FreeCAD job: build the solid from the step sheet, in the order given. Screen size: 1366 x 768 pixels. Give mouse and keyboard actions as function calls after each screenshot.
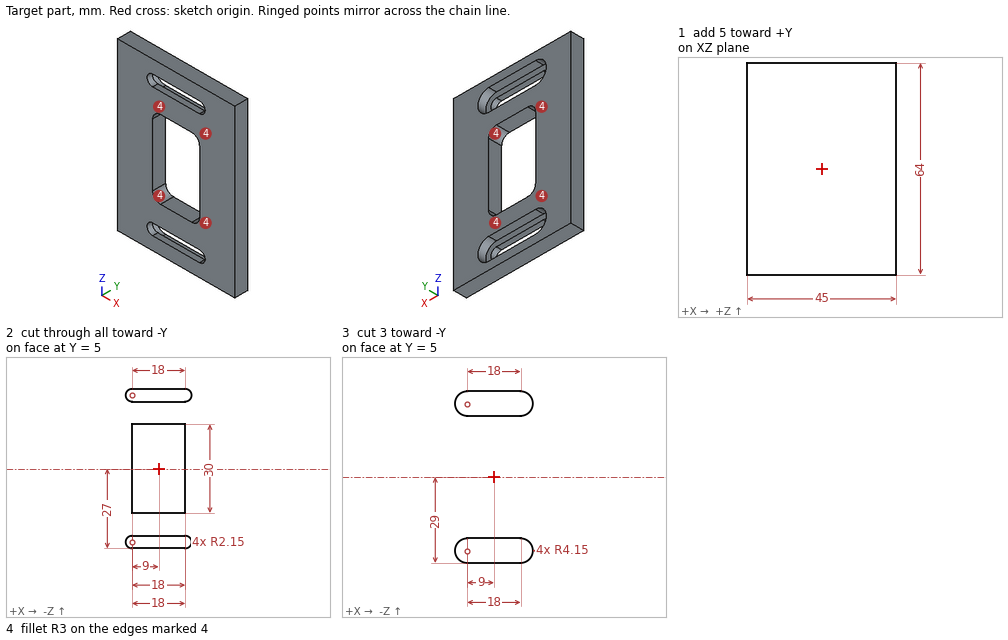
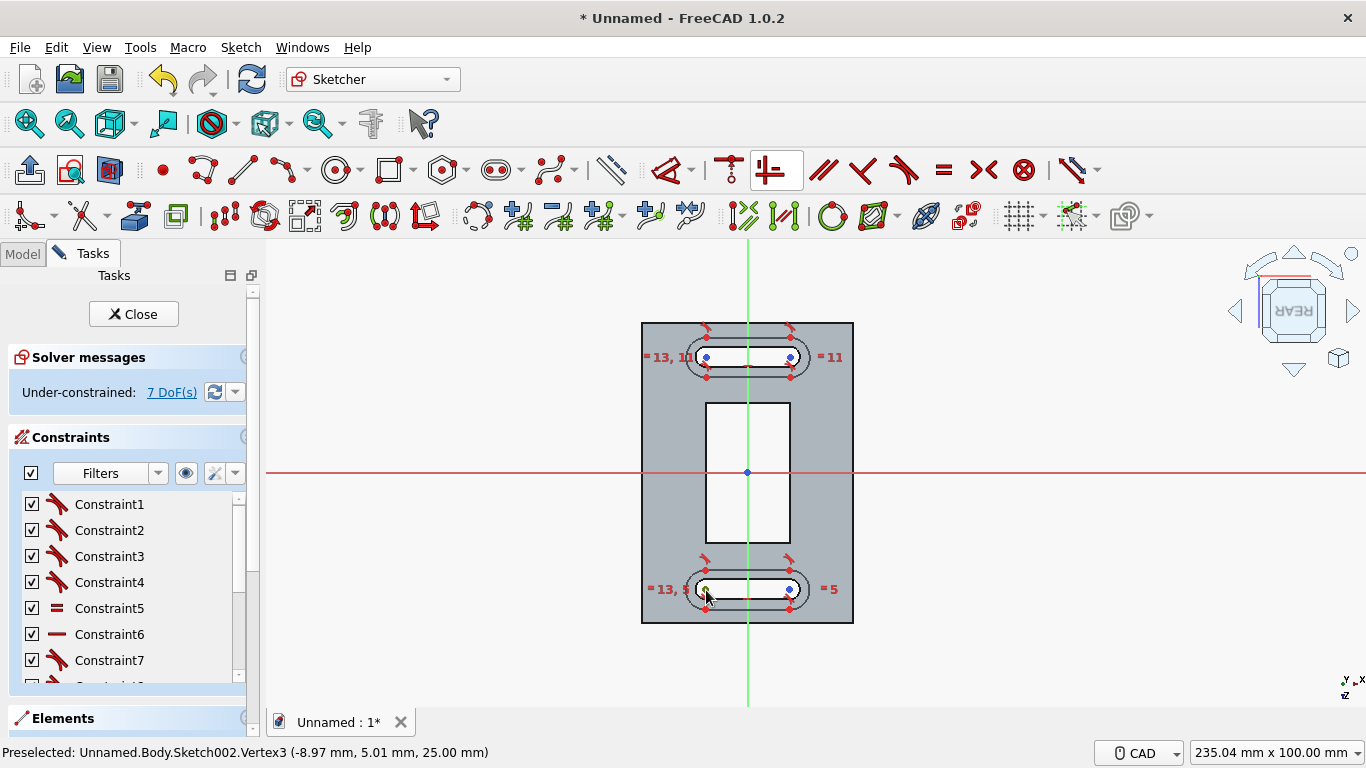
click(706, 358)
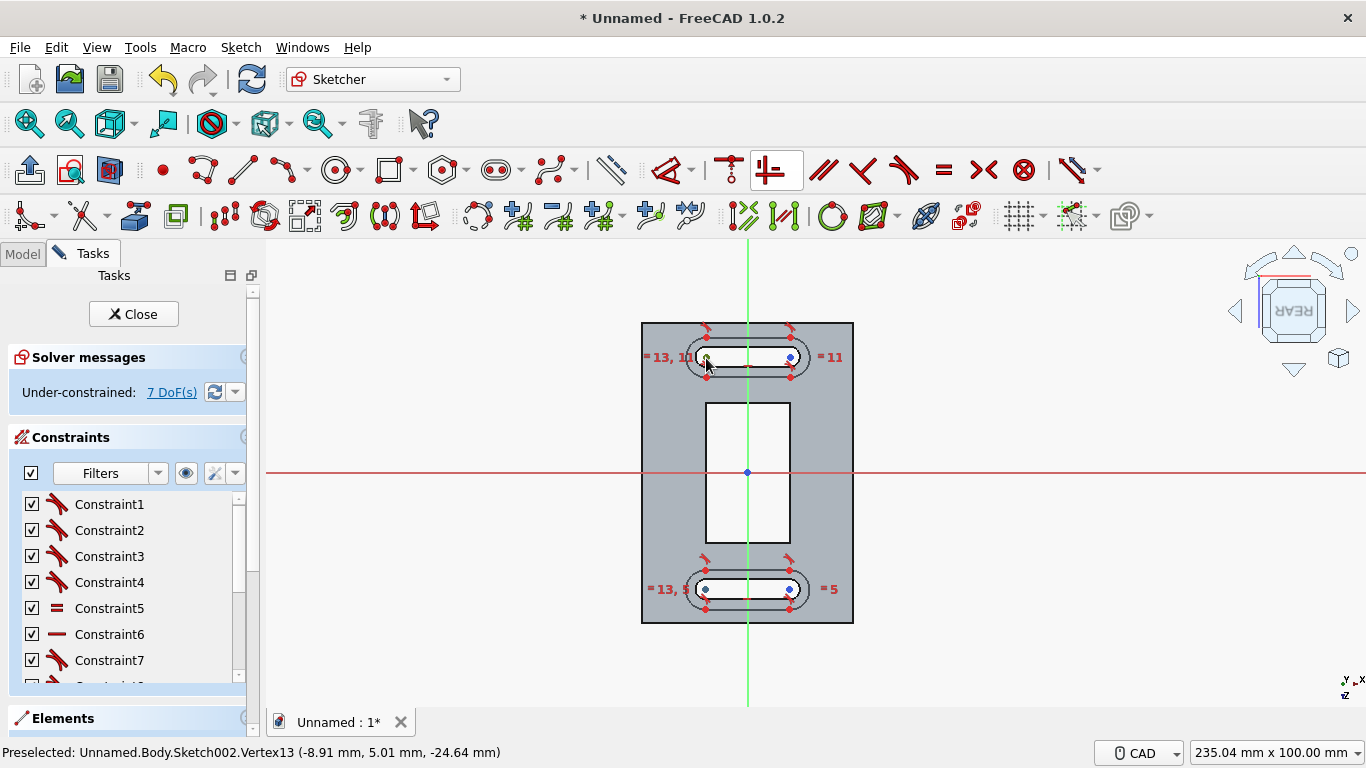
click(359, 473)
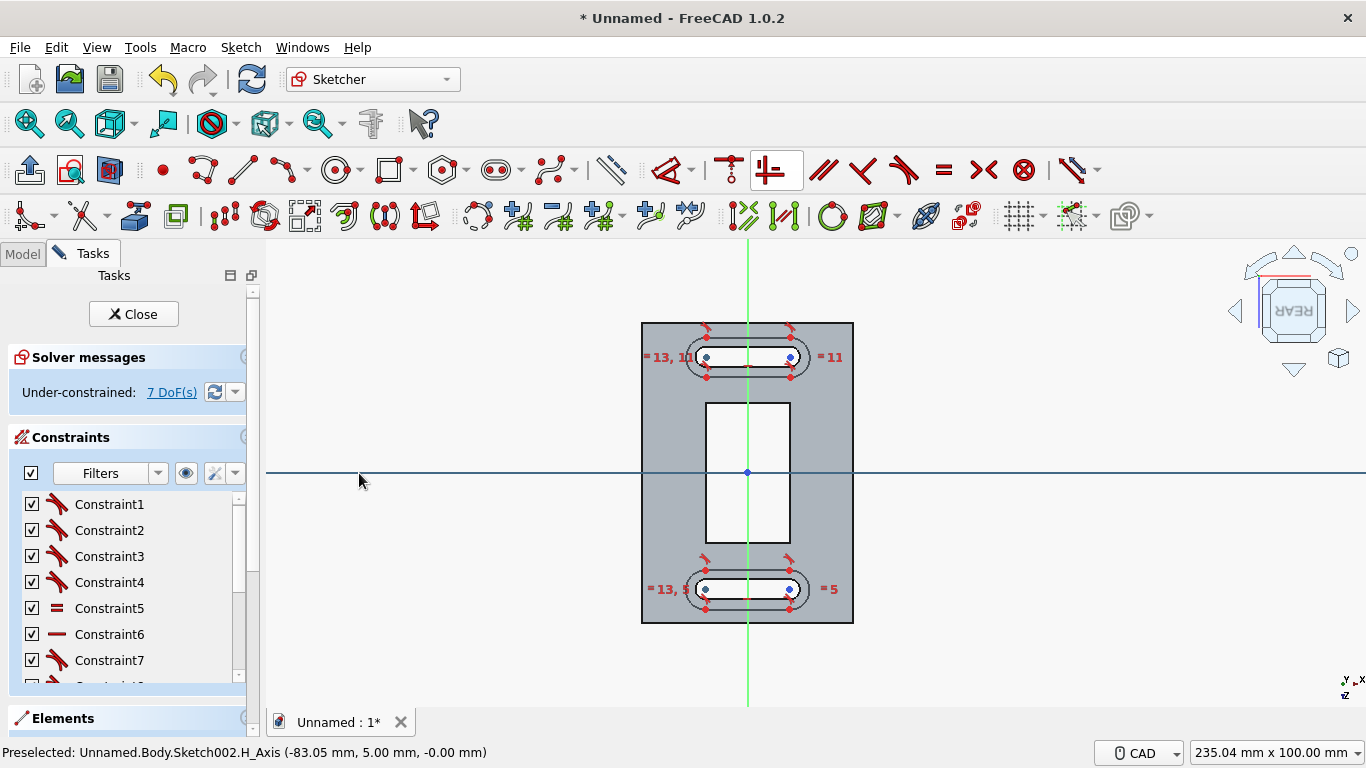
click(984, 170)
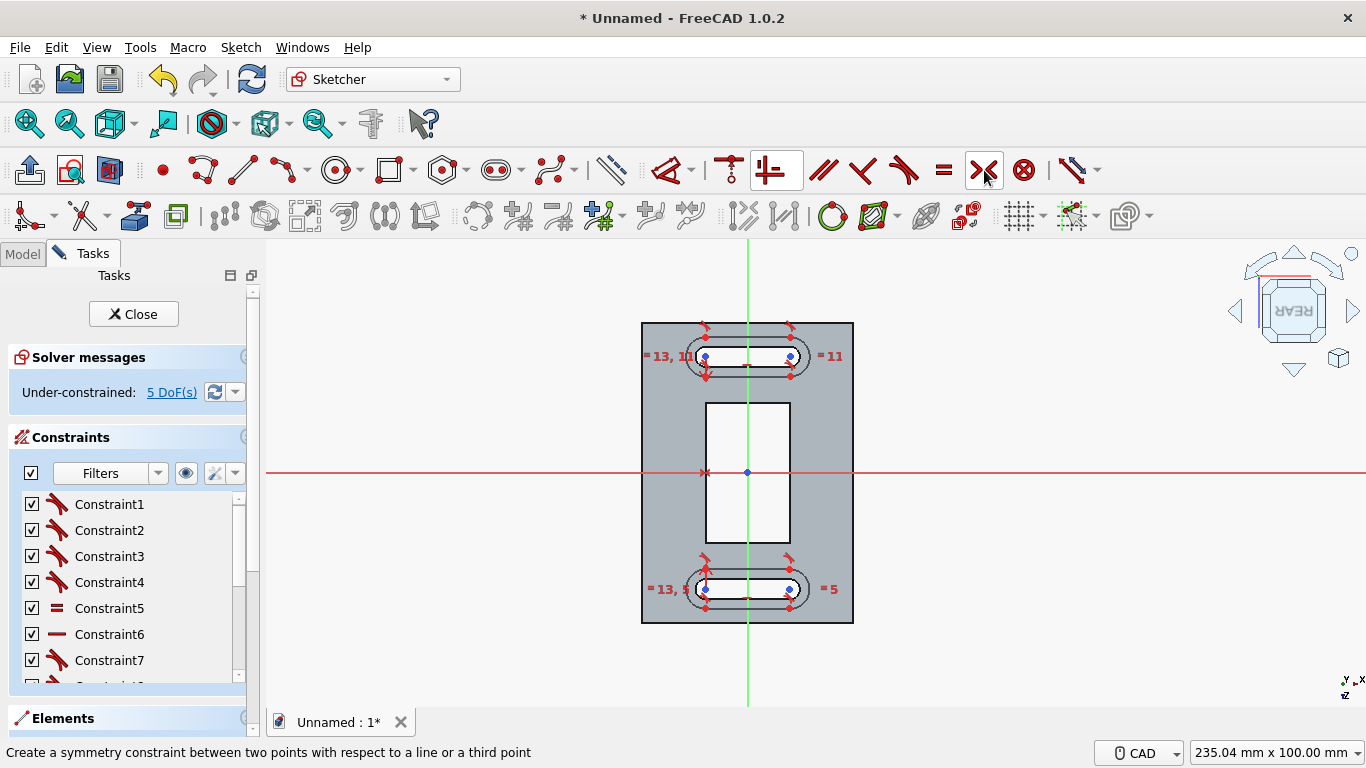
click(666, 170)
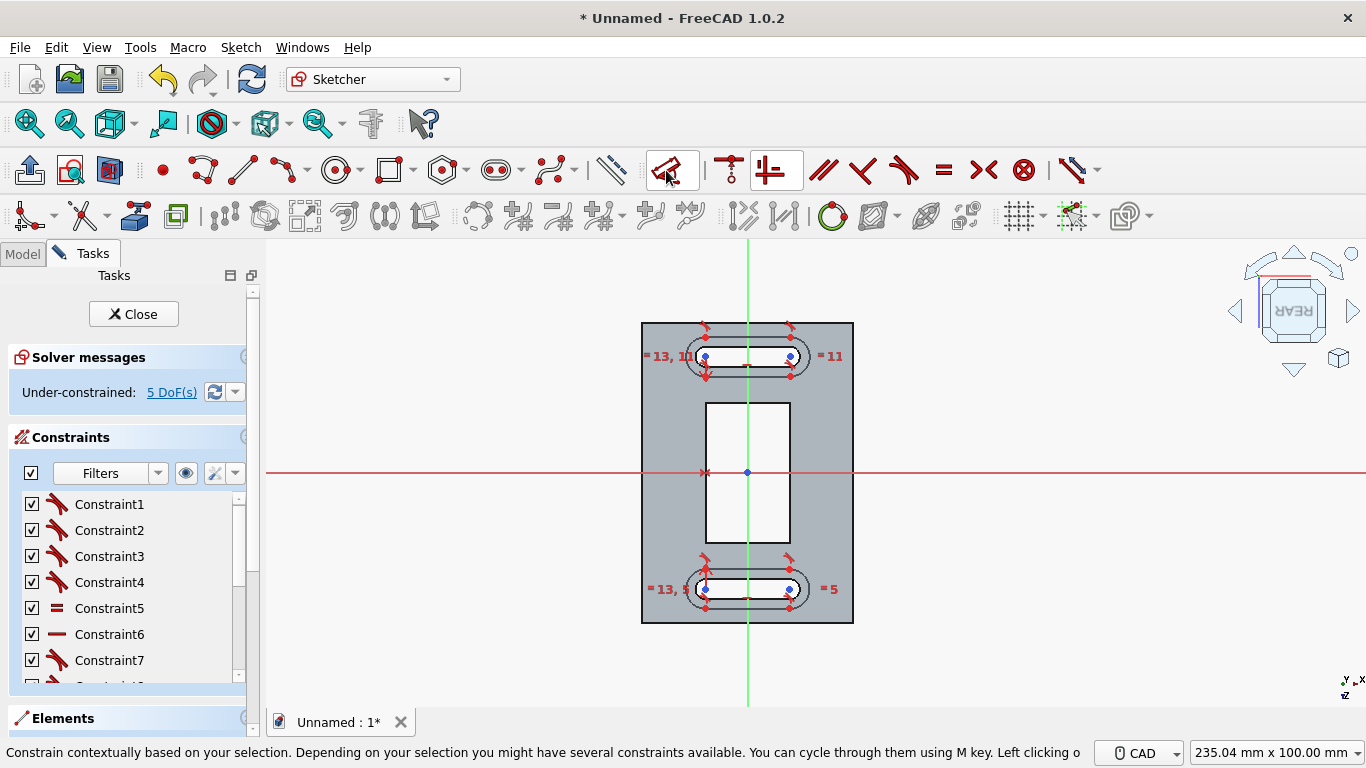
scroll(690, 578, up, 4)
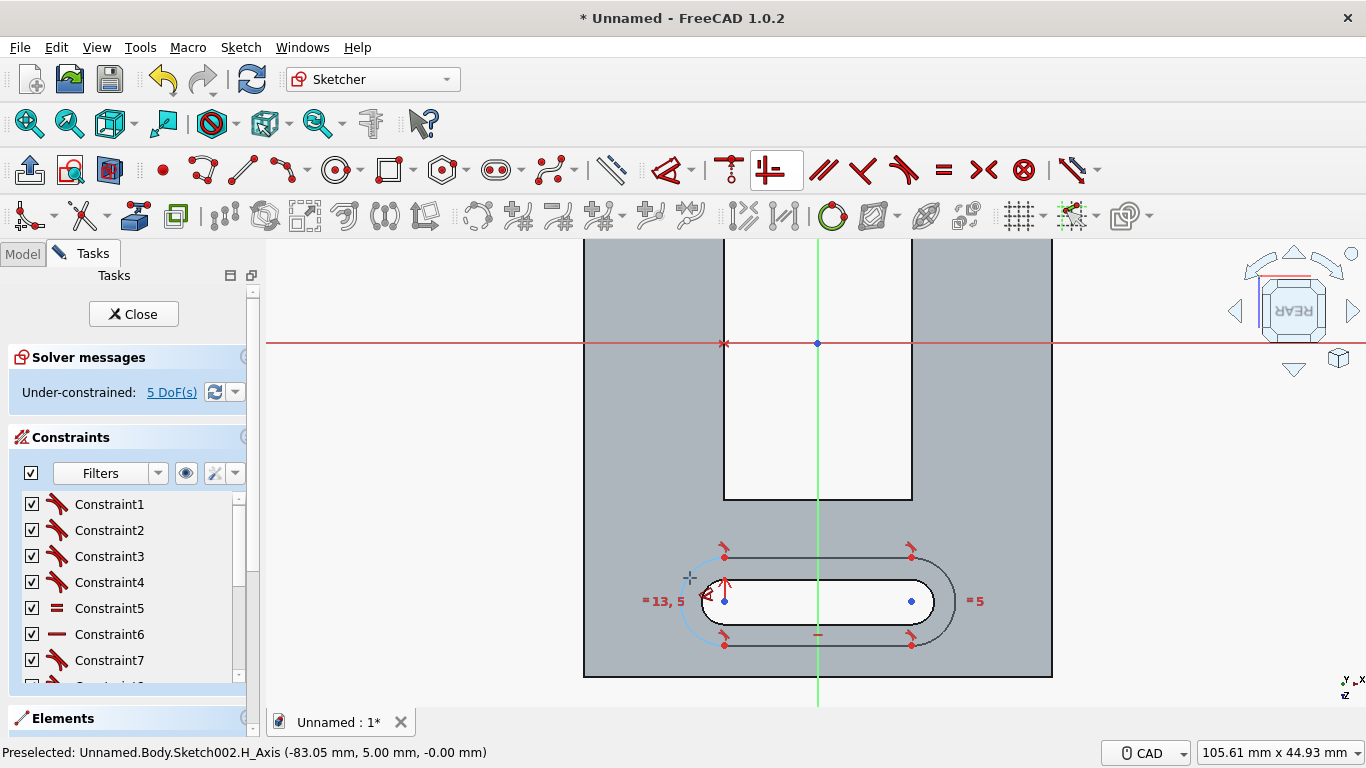
click(689, 576)
click(663, 557)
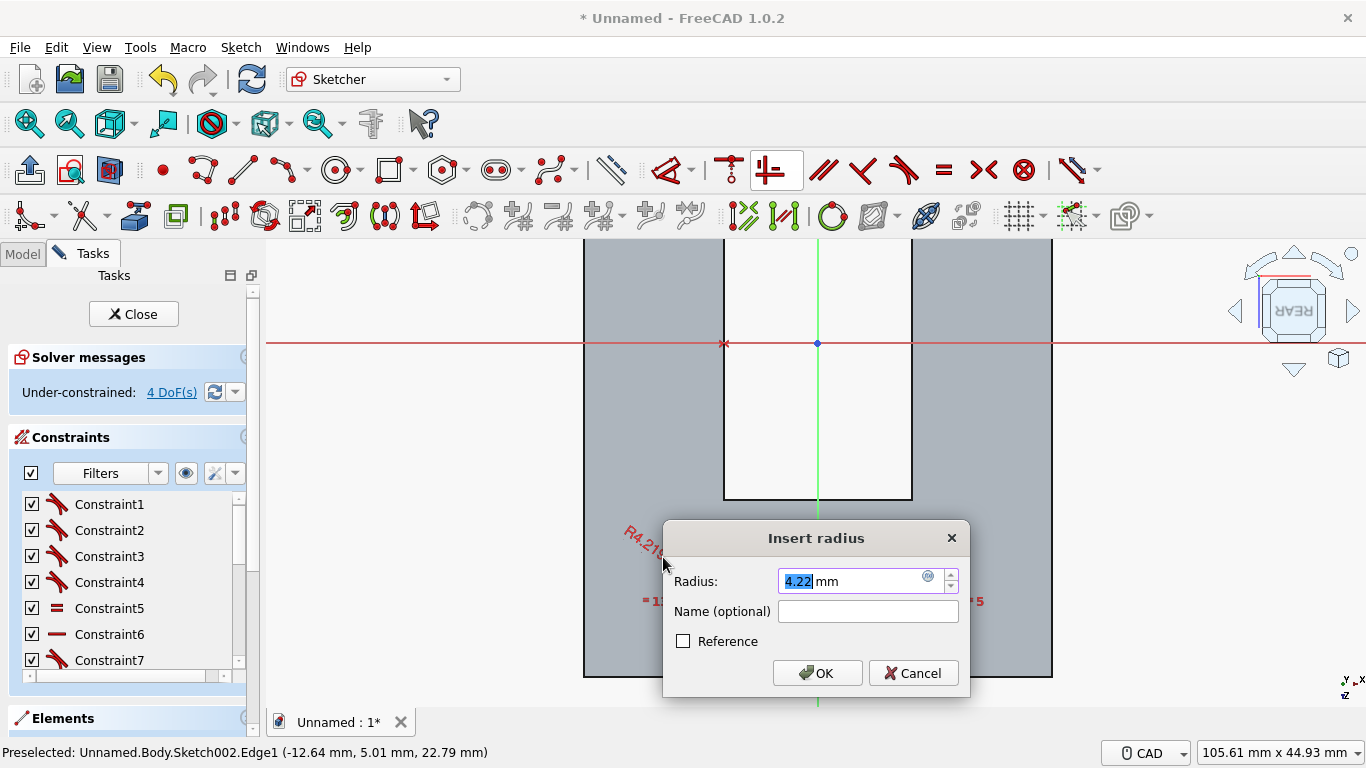
text(4.15)
key(Return)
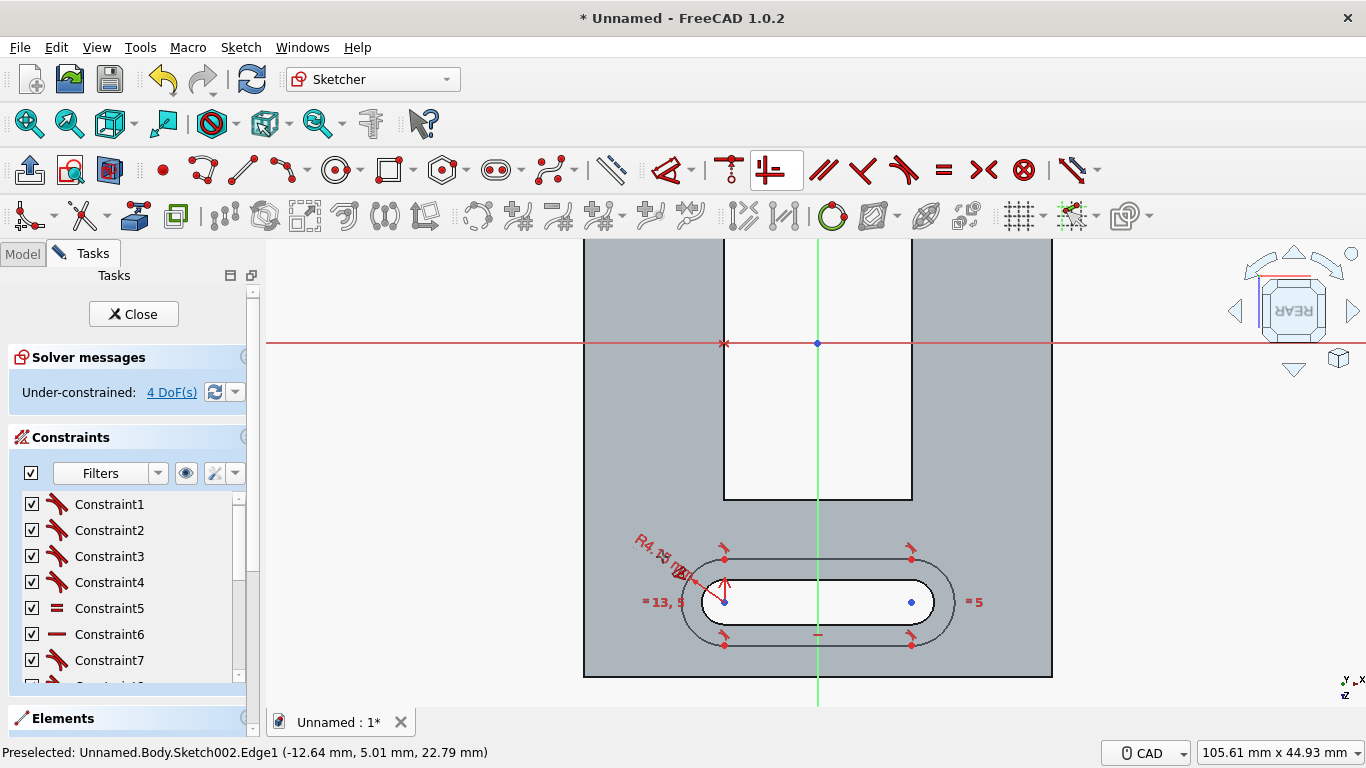
click(781, 559)
click(775, 593)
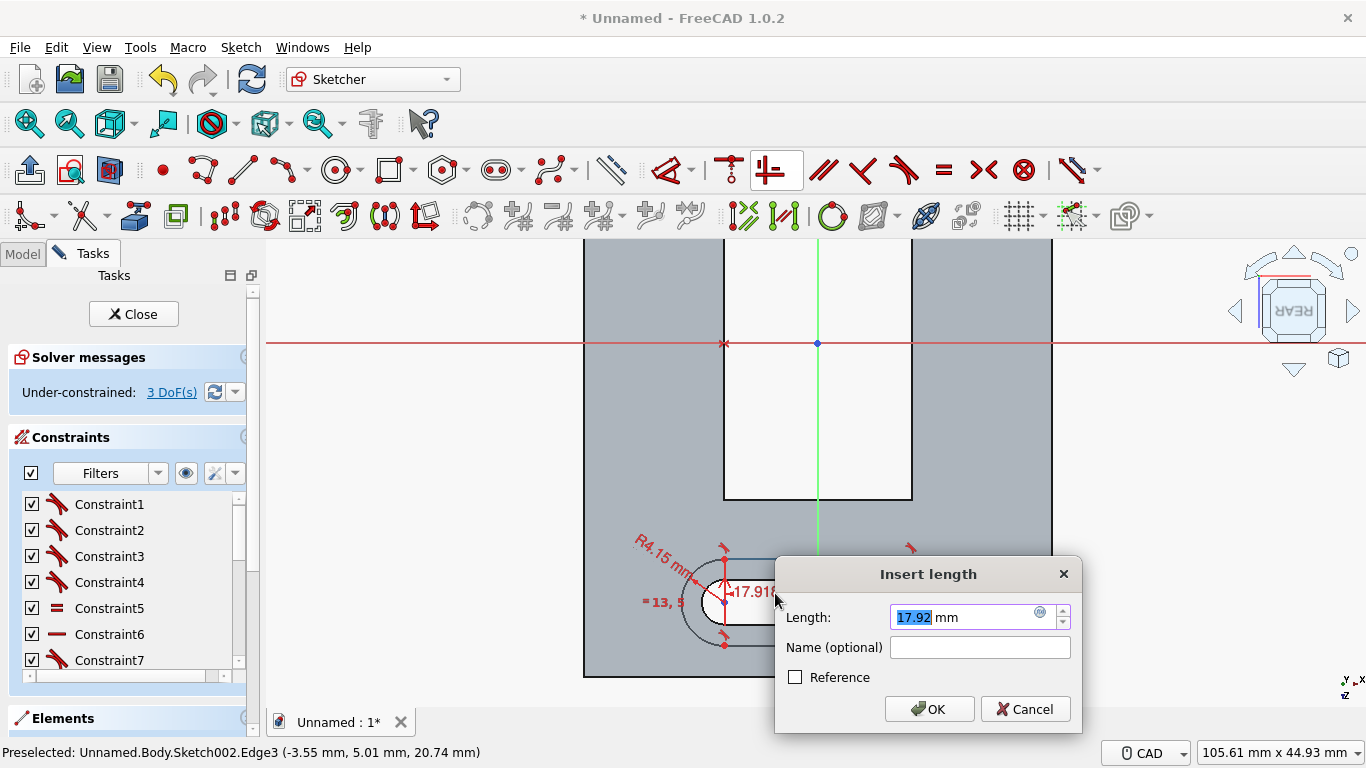
text(18)
key(Return)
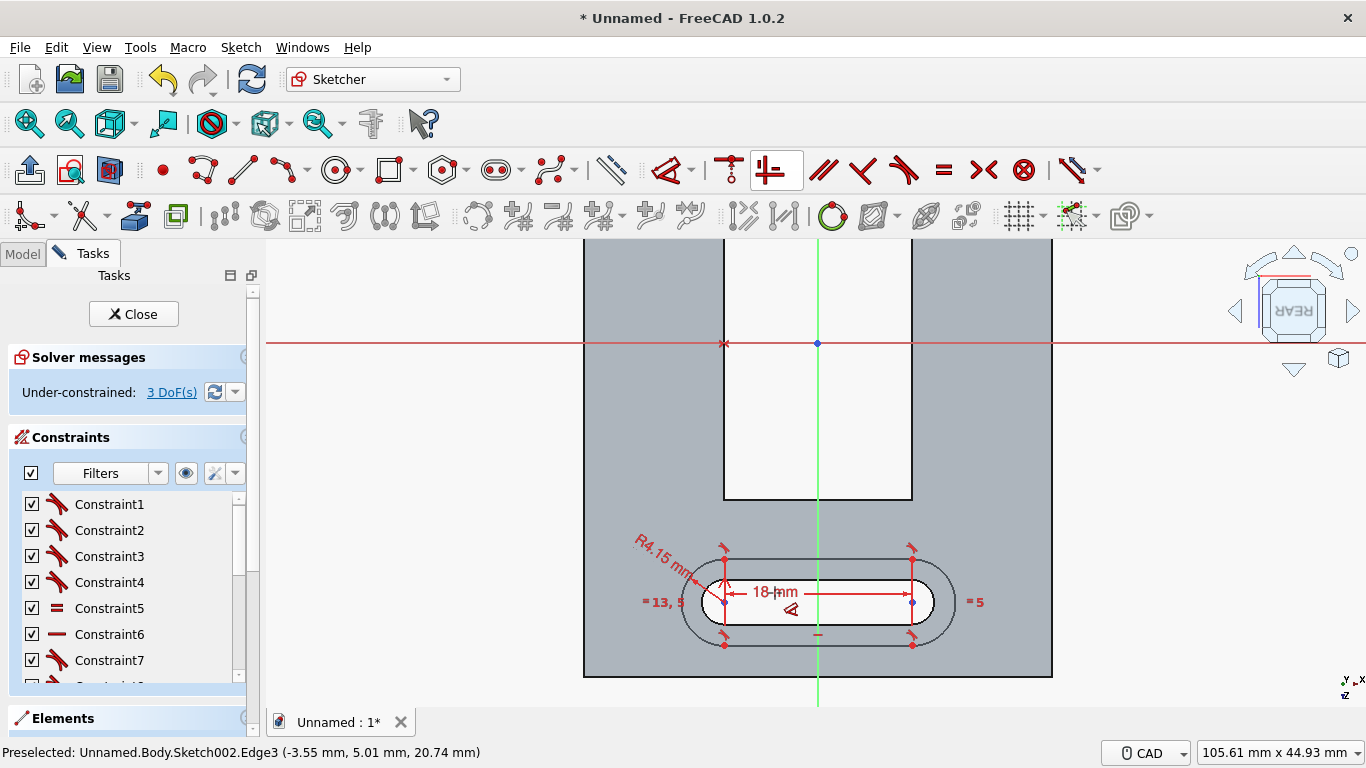
scroll(690, 579, down, 4)